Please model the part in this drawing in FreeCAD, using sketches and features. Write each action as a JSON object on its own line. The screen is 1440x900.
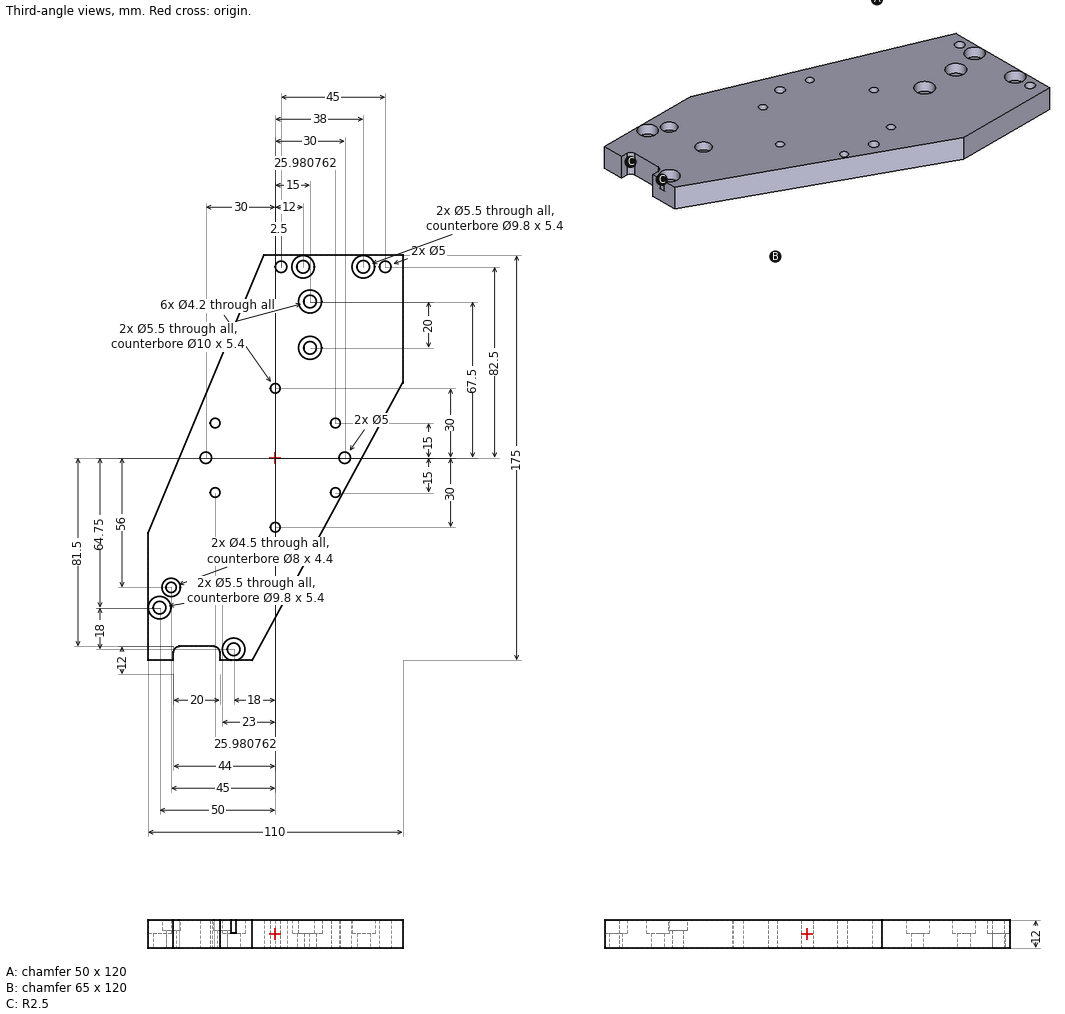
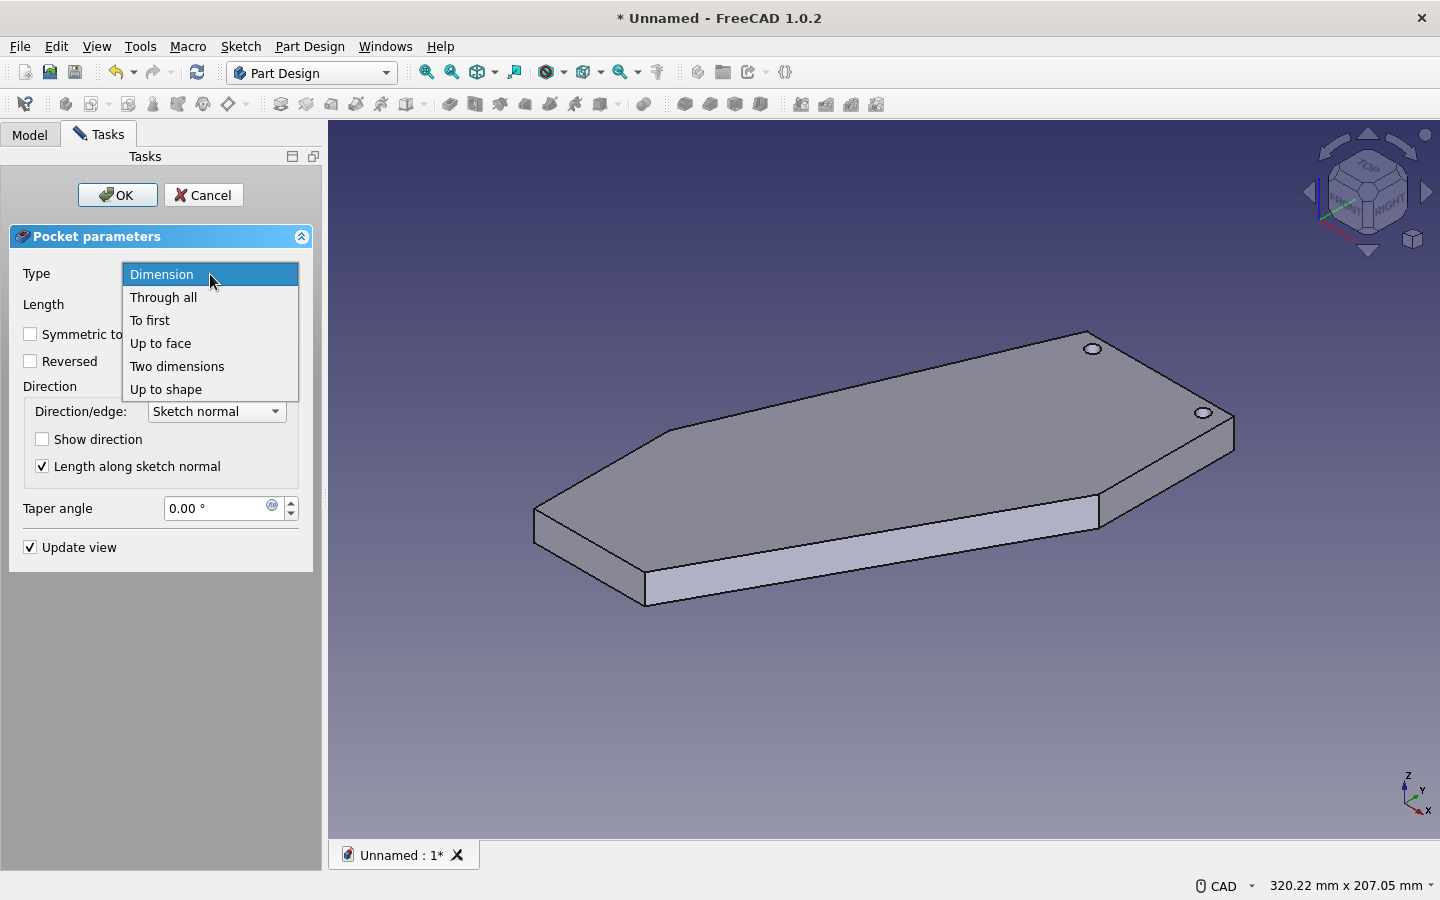
{"action": "left_click", "coordinate": [208, 298]}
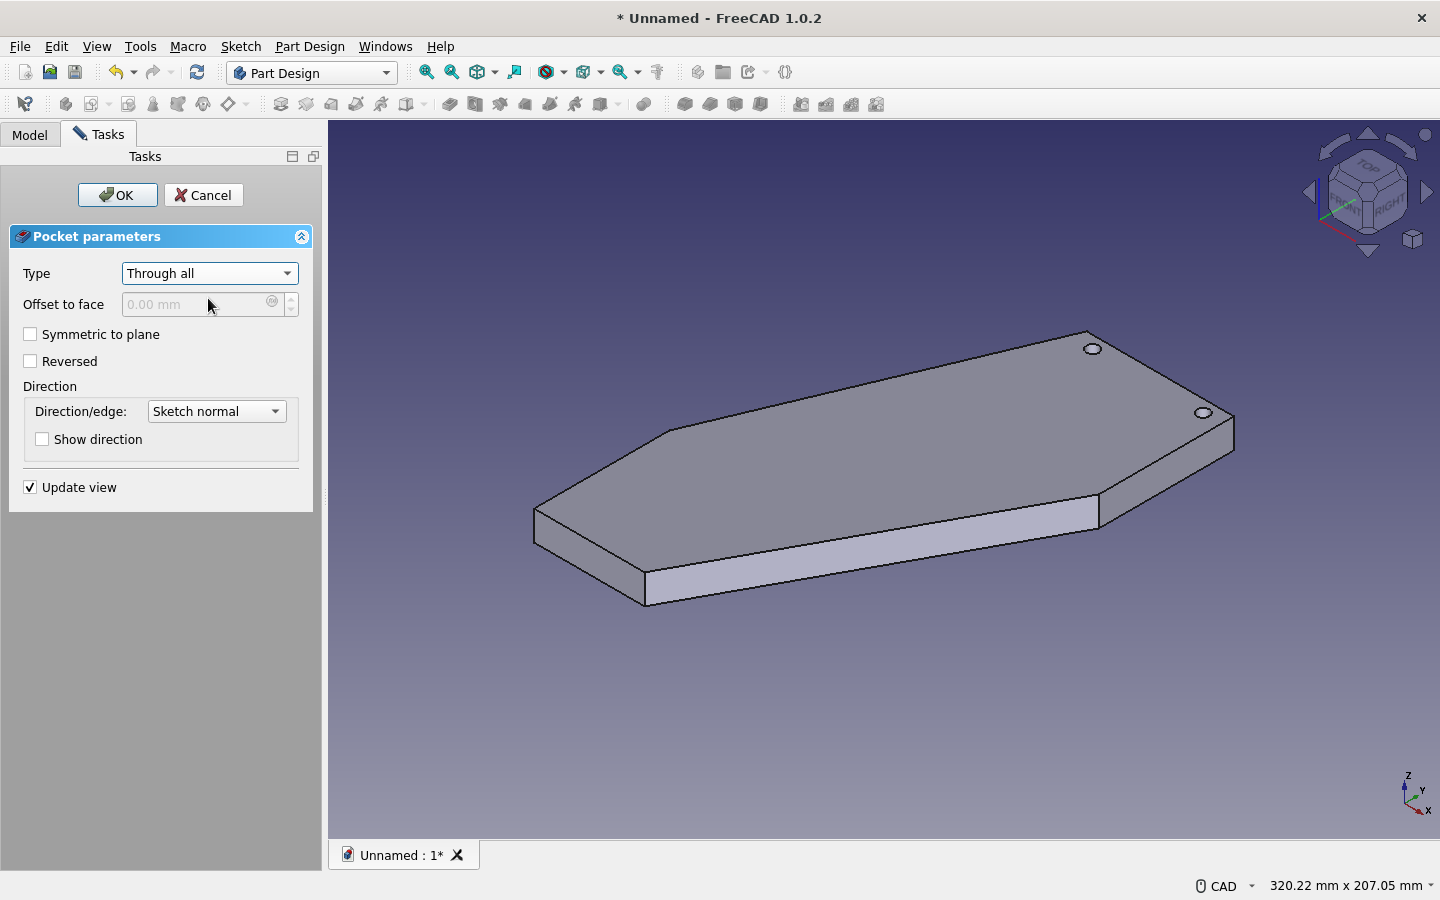
{"action": "left_click", "coordinate": [118, 195]}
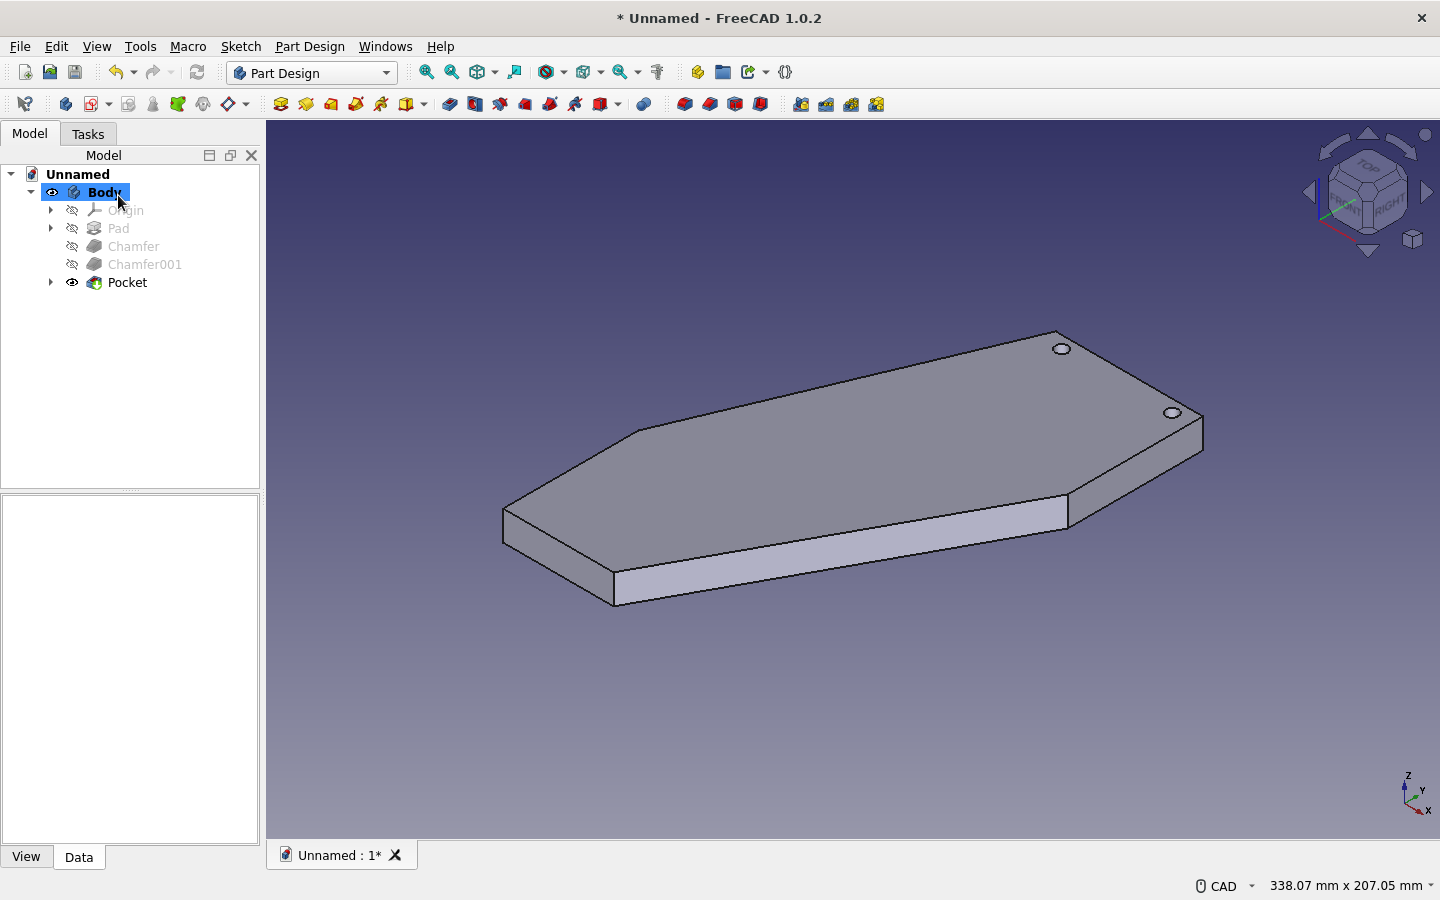
{"action": "left_click", "coordinate": [753, 475]}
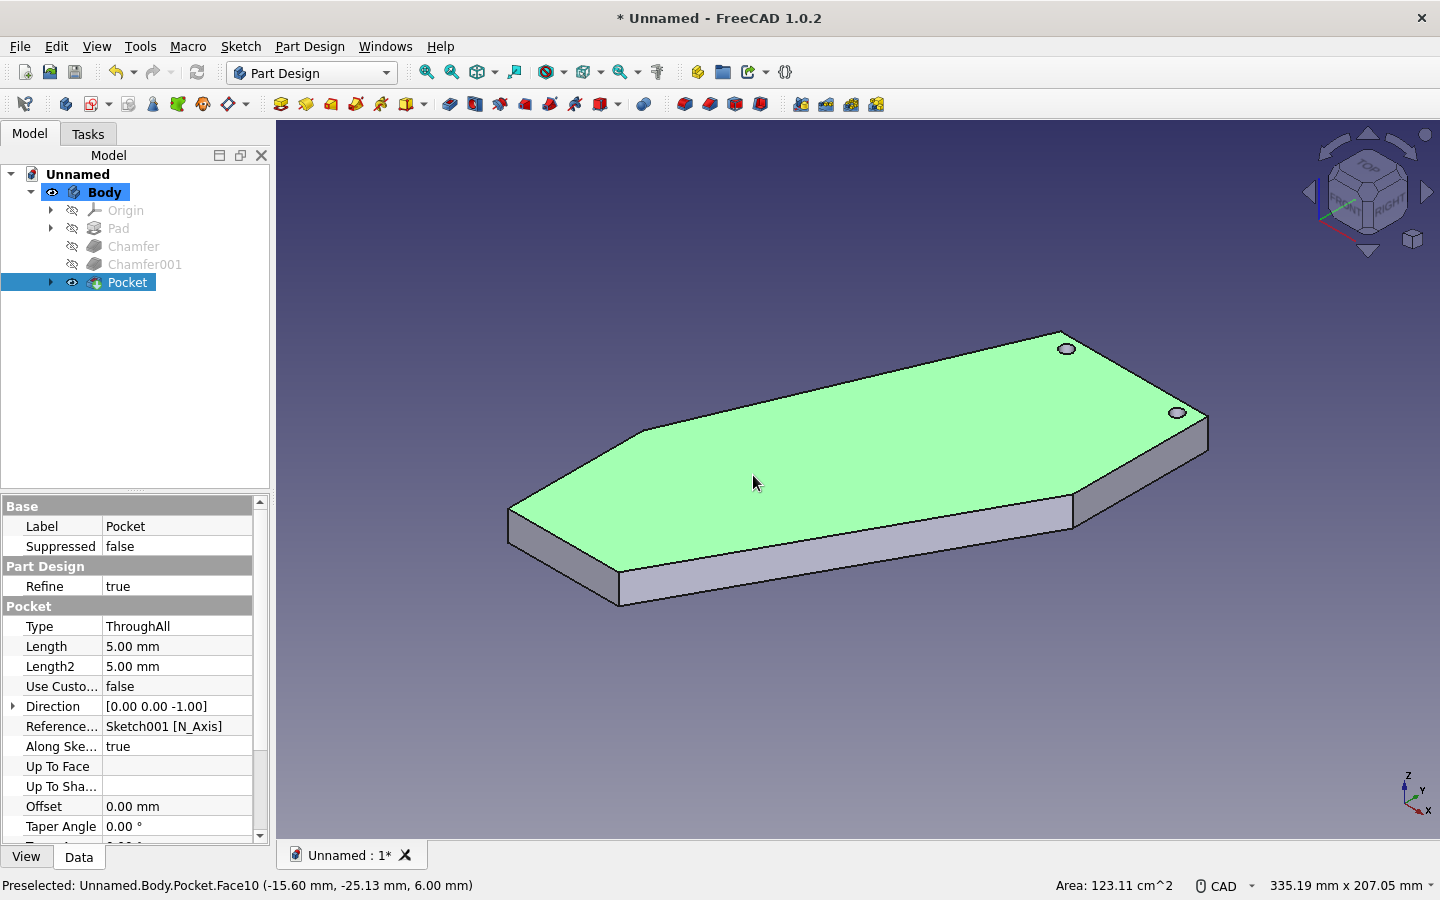
{"action": "left_click", "coordinate": [90, 104]}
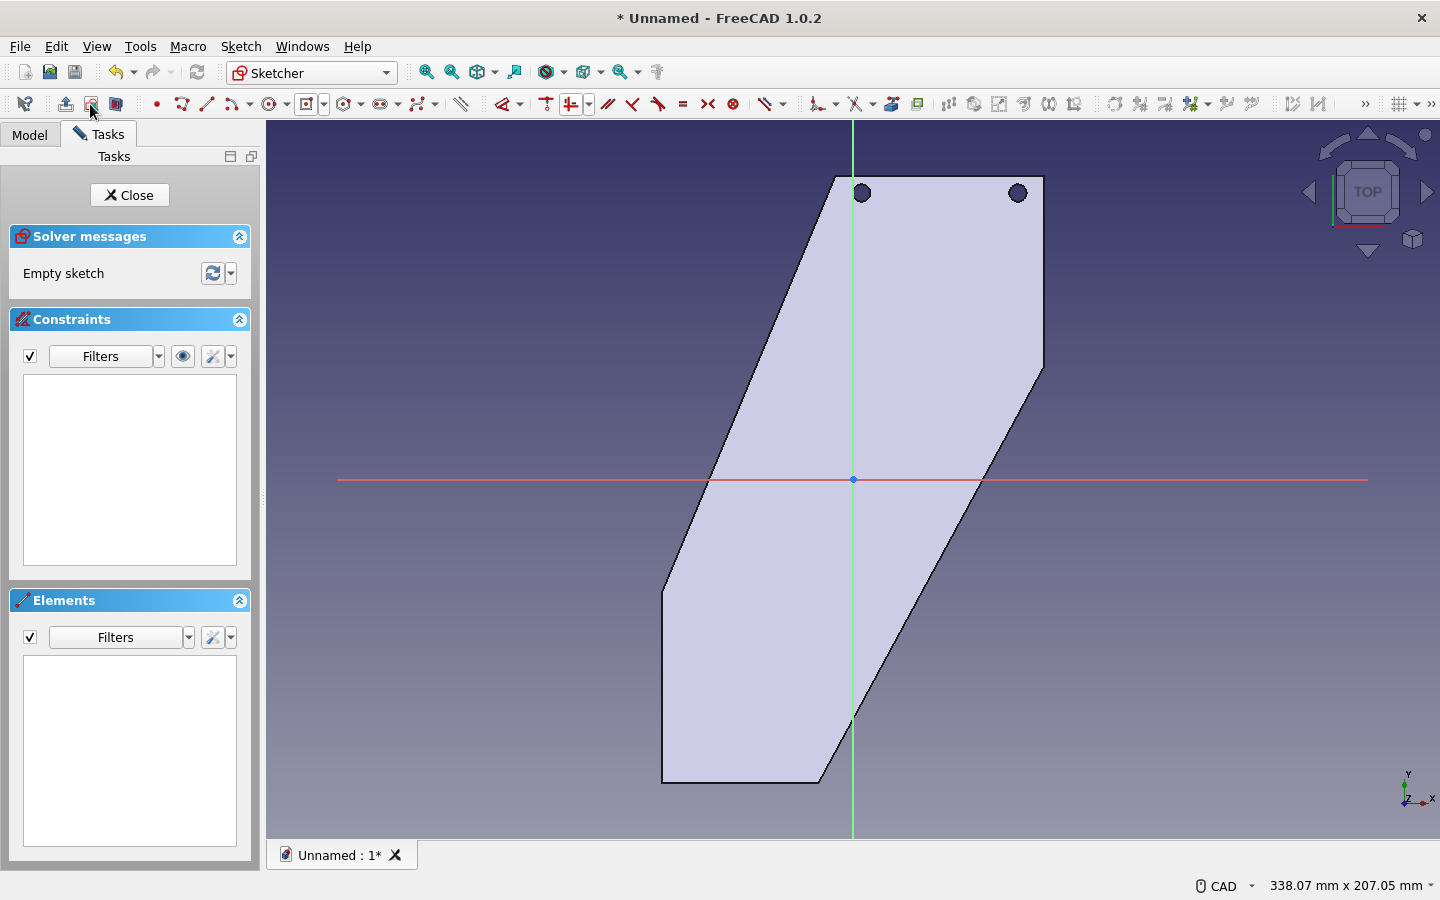
{"action": "scroll", "coordinate": [909, 479], "scroll_direction": "up", "scroll_amount": 4}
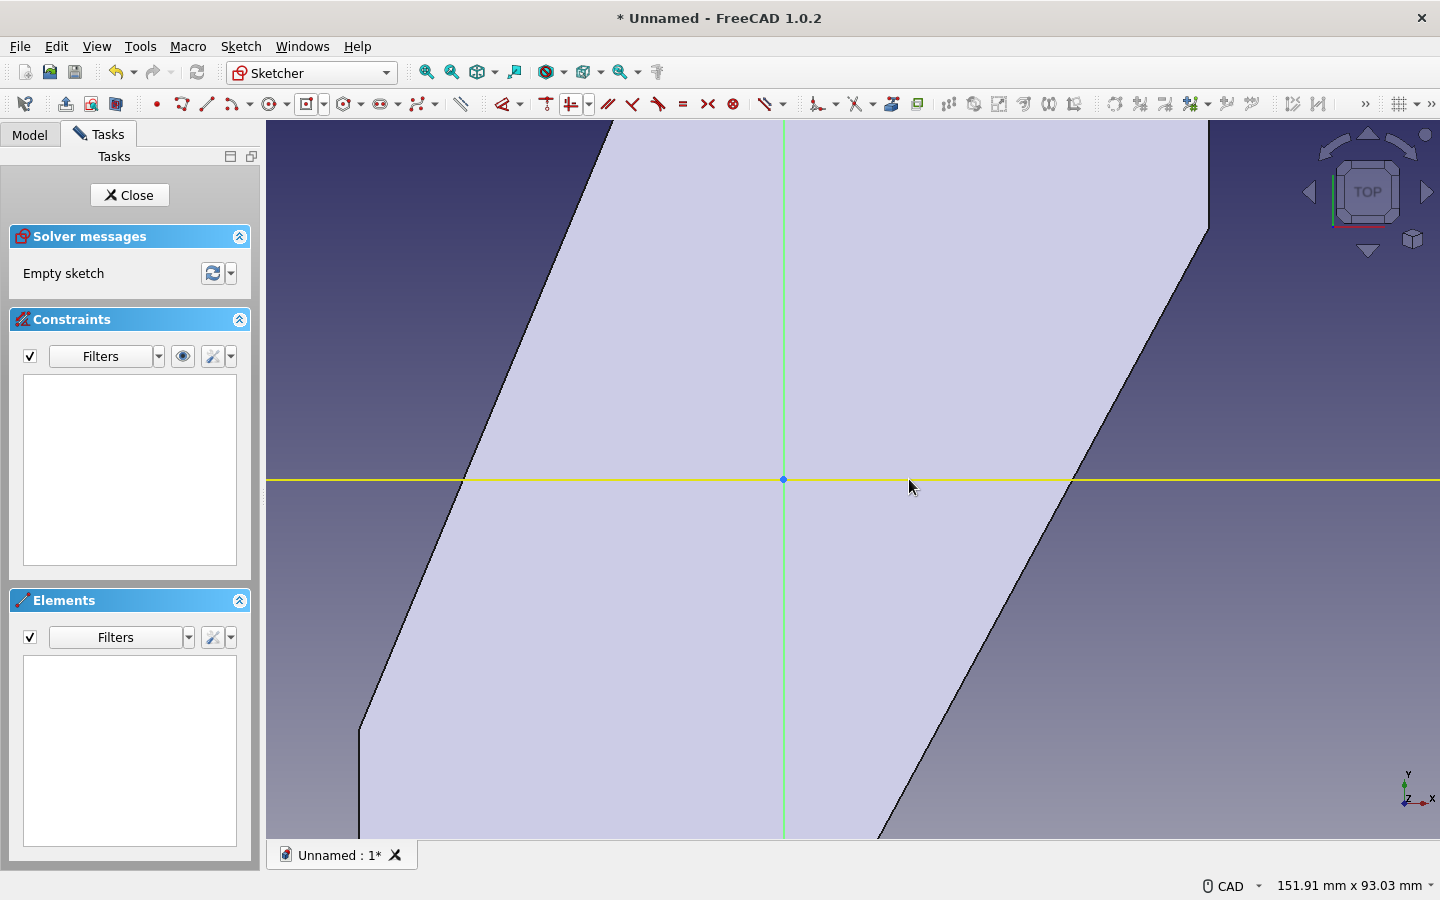
{"action": "key", "text": "g c"}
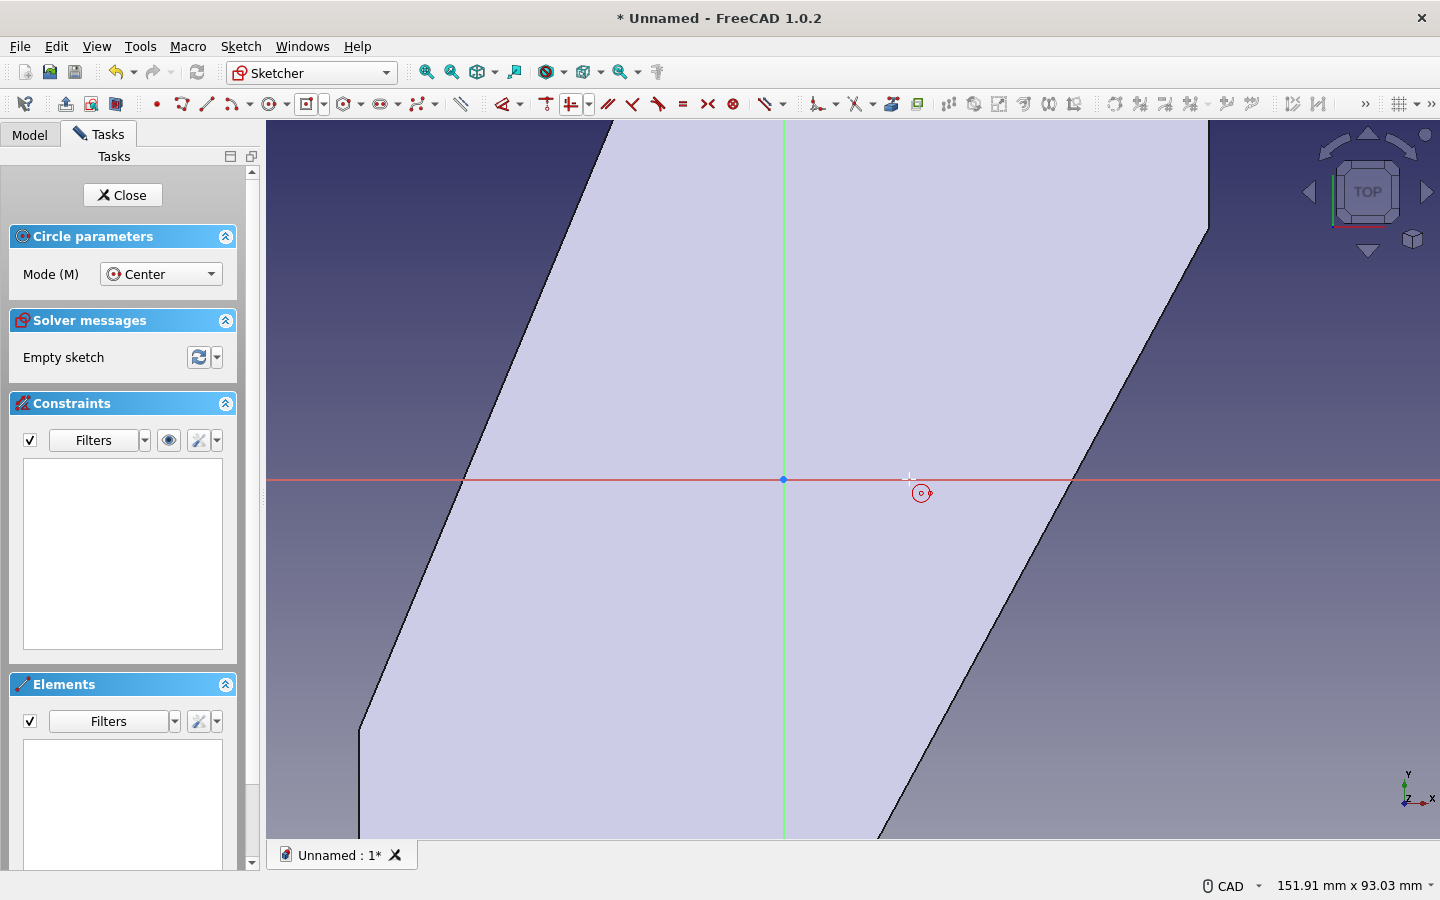
{"action": "scroll", "coordinate": [784, 248], "scroll_direction": "up", "scroll_amount": 2}